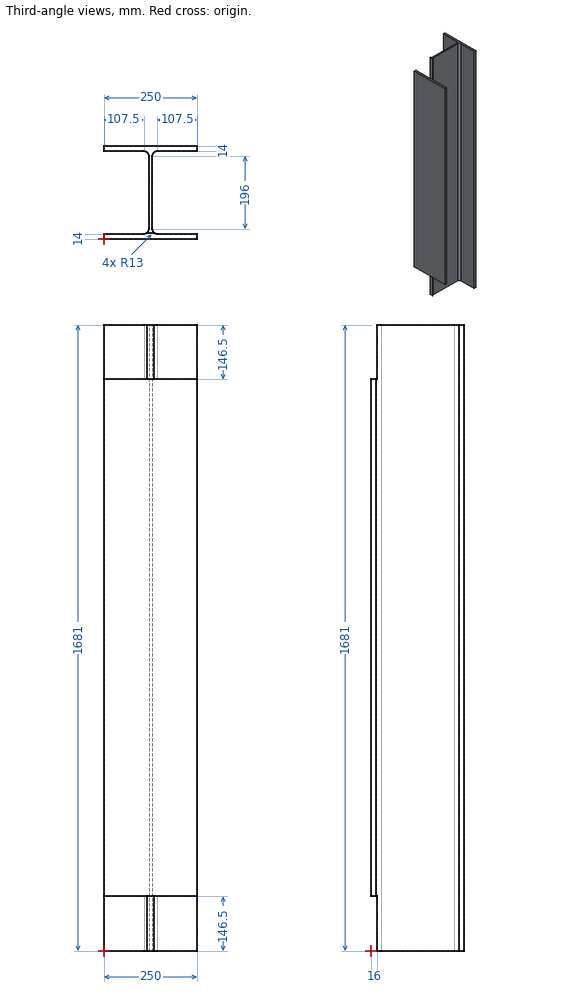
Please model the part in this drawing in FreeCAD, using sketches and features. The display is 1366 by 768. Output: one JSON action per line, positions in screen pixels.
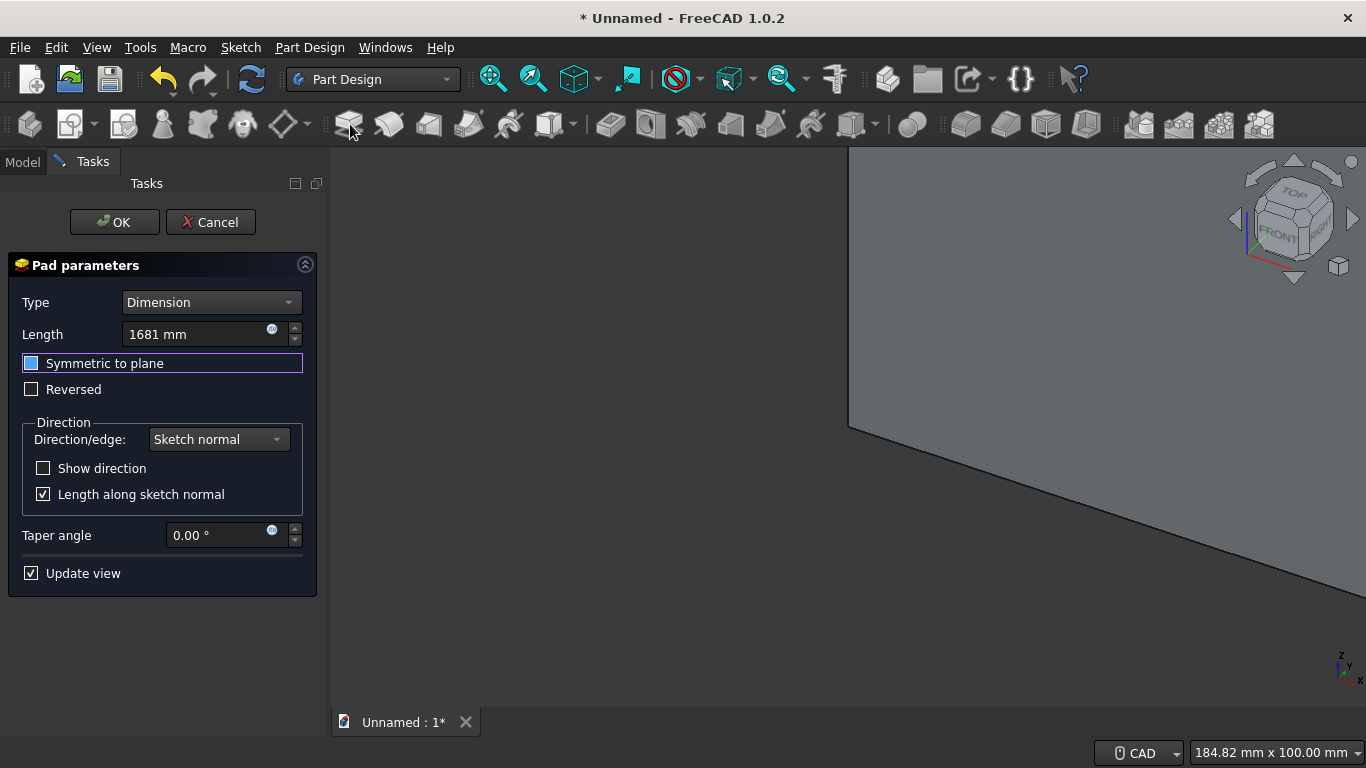
{"action": "left_click", "coordinate": [115, 222]}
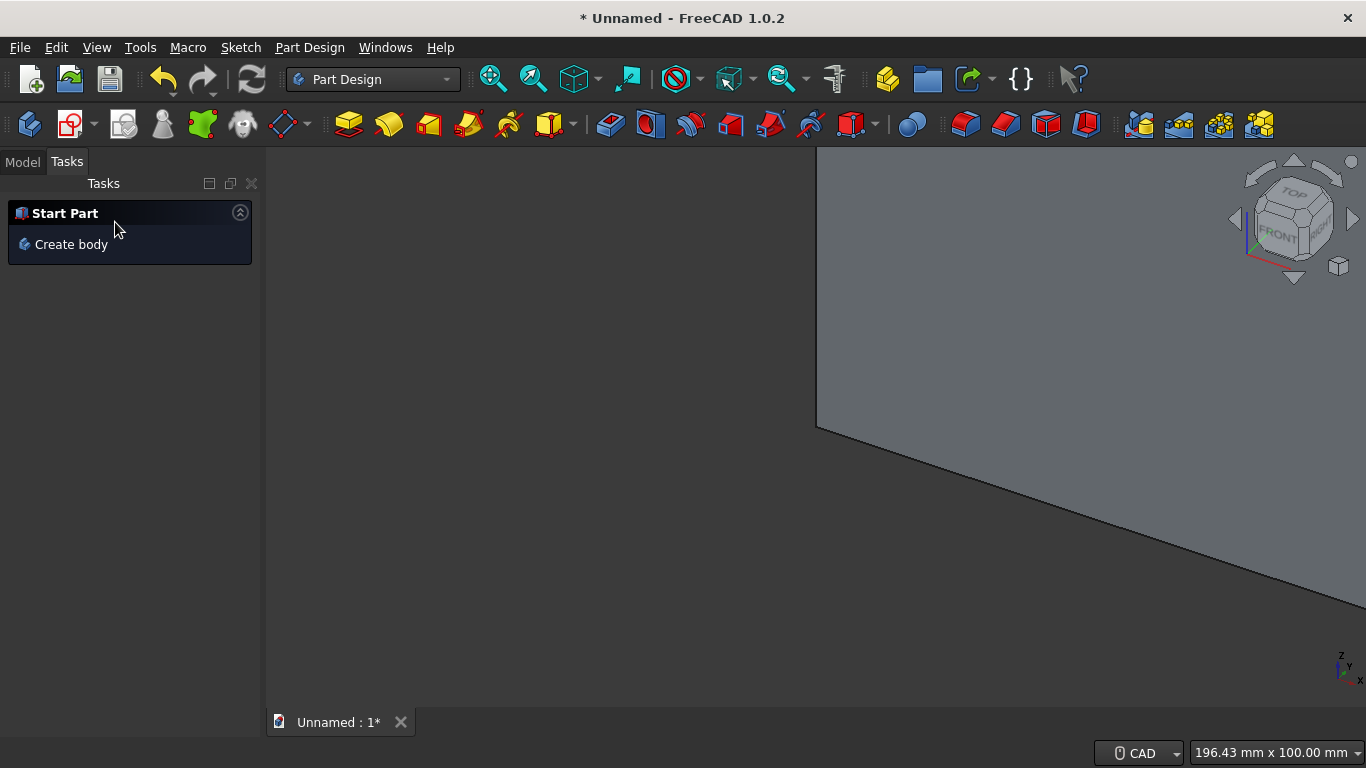
{"action": "left_click", "coordinate": [494, 80]}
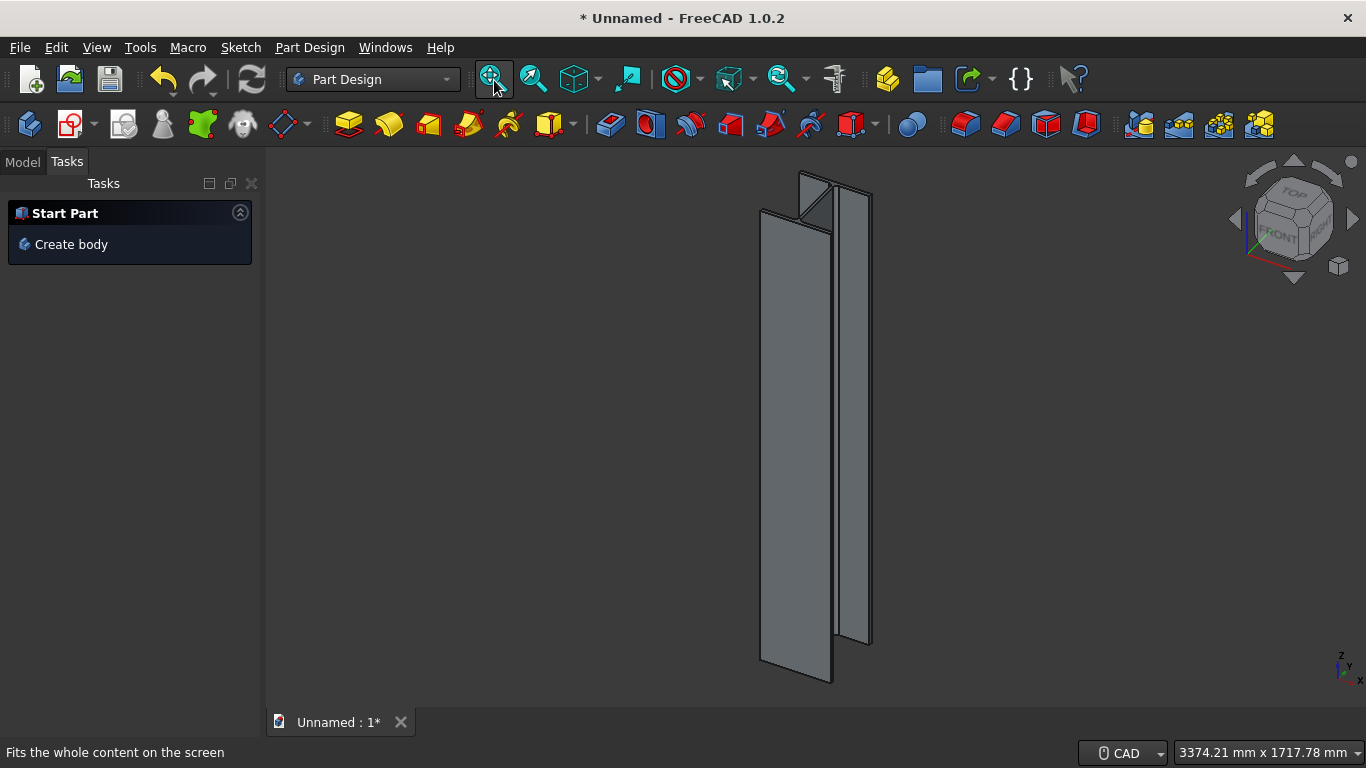
{"action": "left_click", "coordinate": [796, 318]}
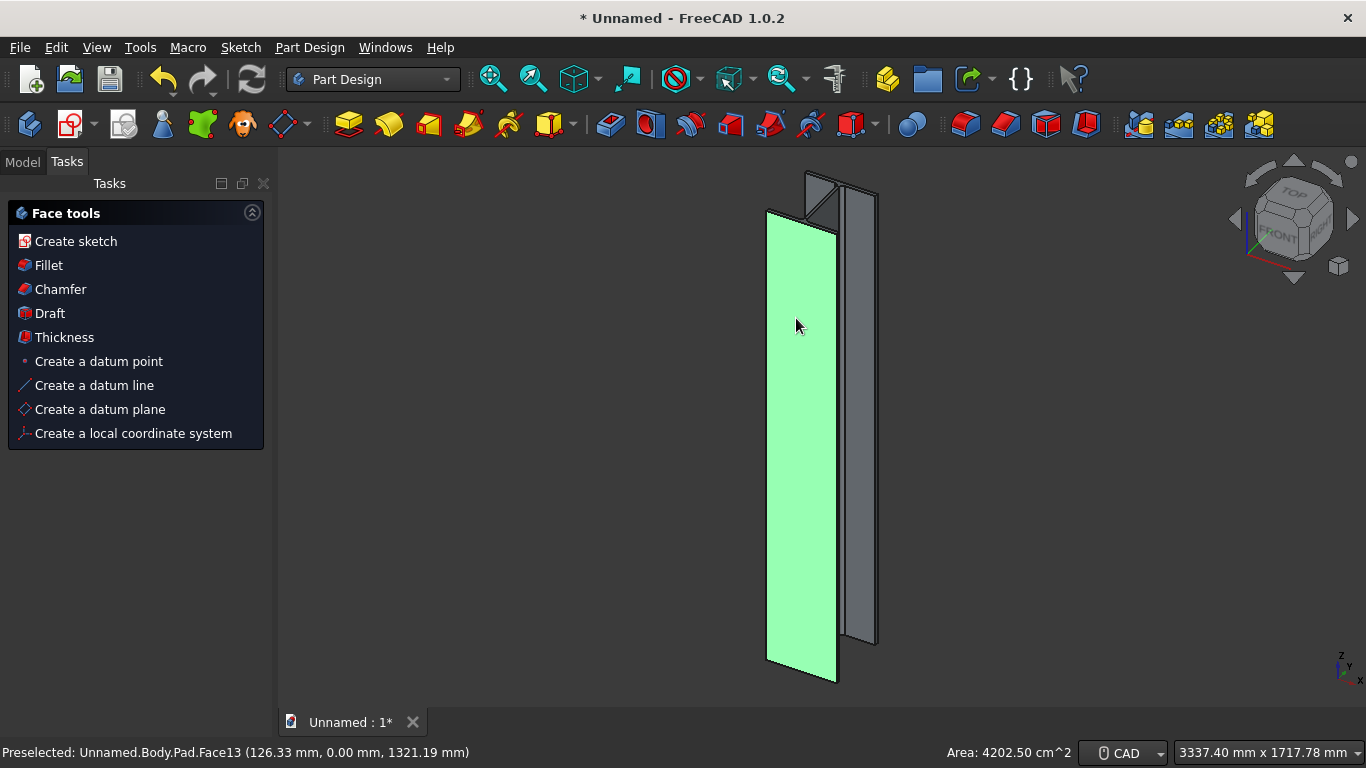
{"action": "left_click", "coordinate": [70, 124]}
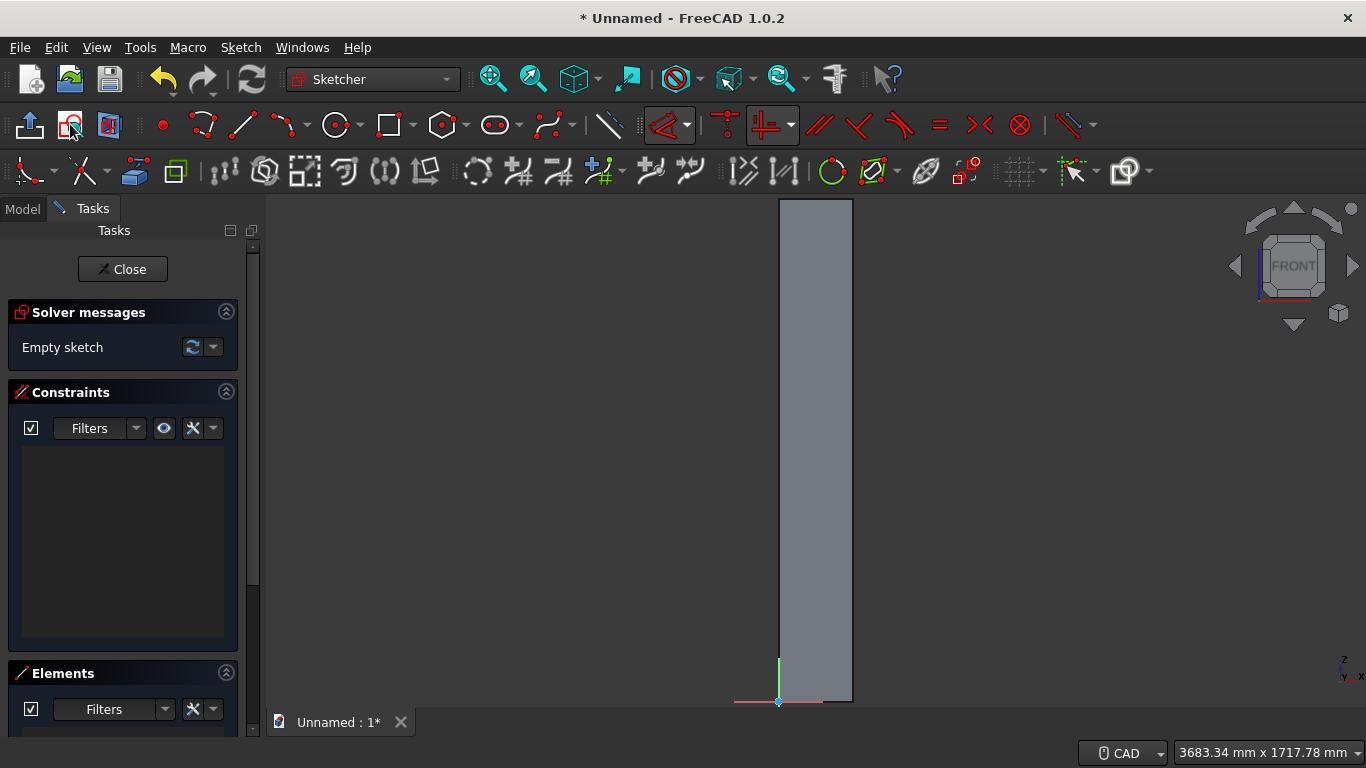
{"action": "scroll", "coordinate": [608, 451], "scroll_direction": "down", "scroll_amount": 2}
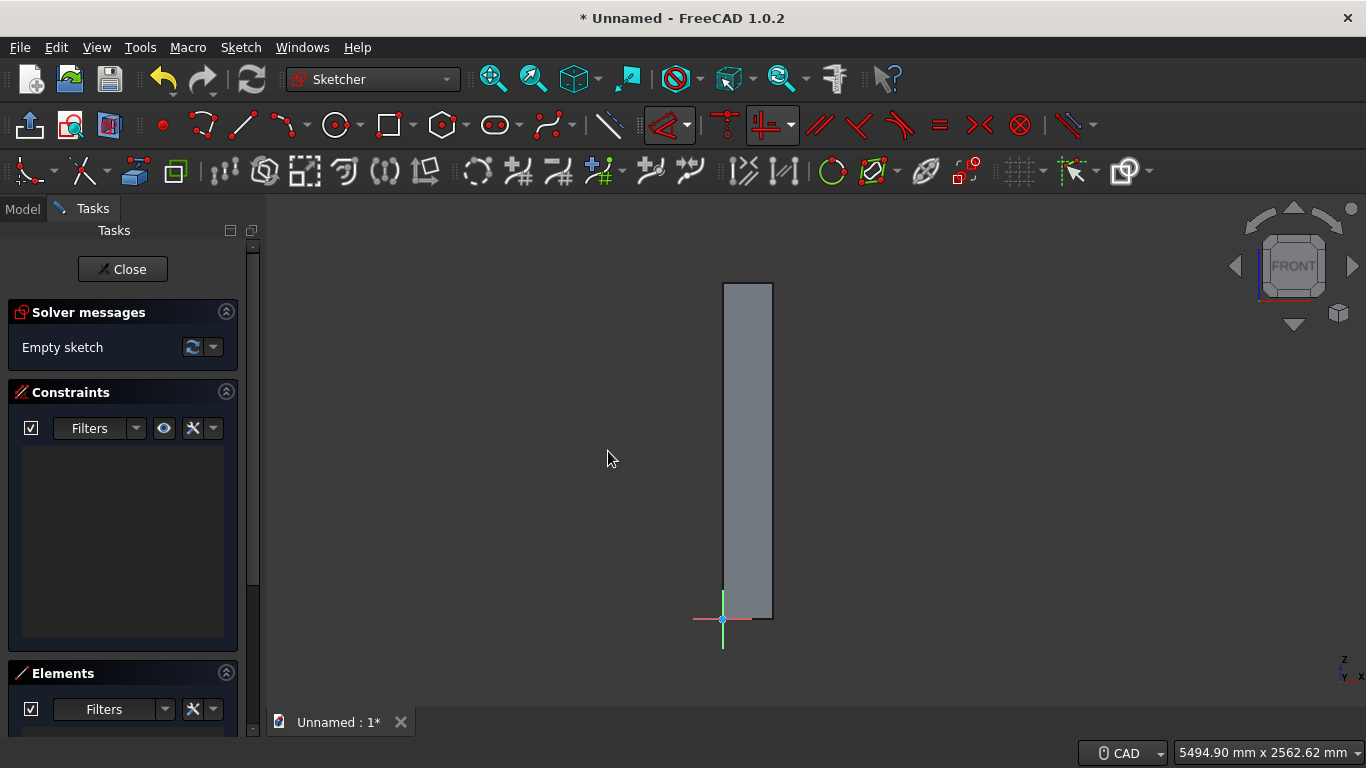
{"action": "left_click", "coordinate": [390, 126]}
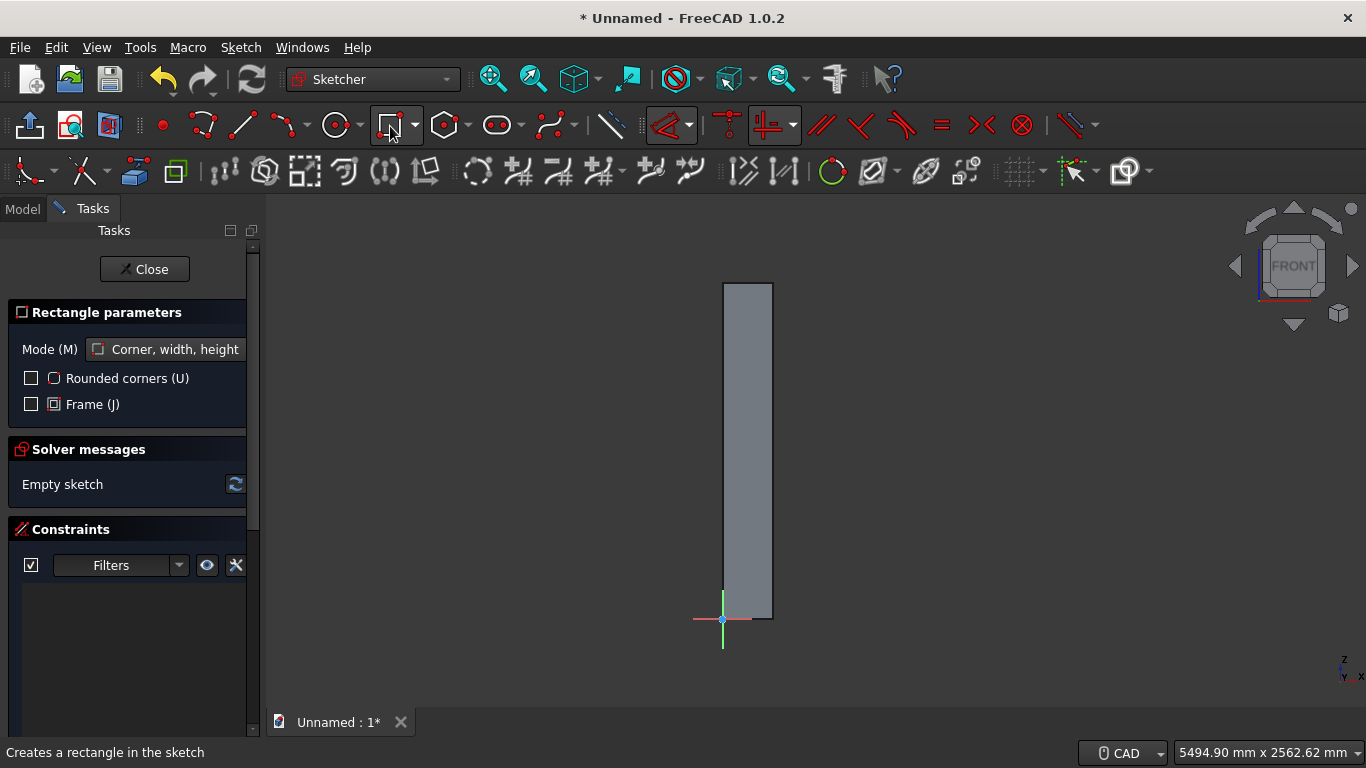
{"action": "left_click", "coordinate": [723, 619]}
{"action": "mouse_move", "coordinate": [773, 590]}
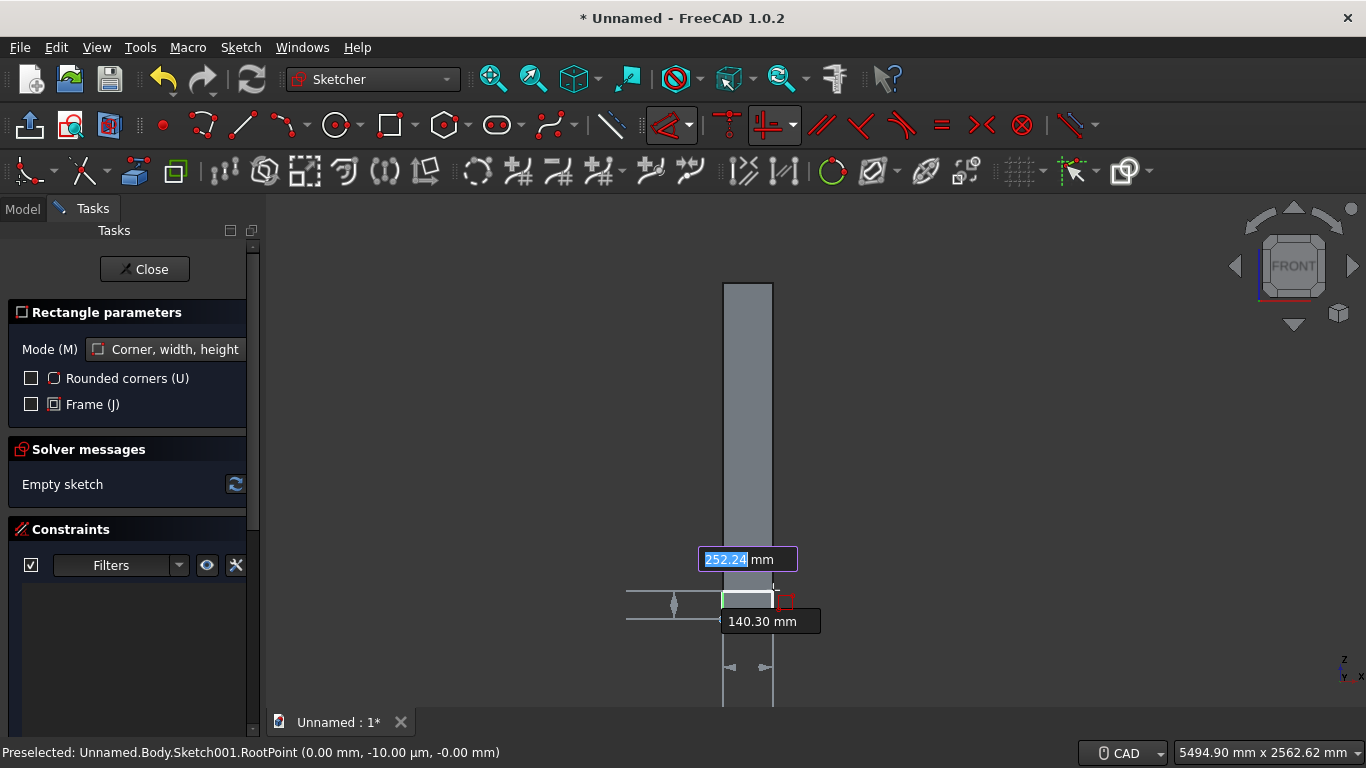
{"action": "type", "text": "250"}
{"action": "key", "text": "Tab"}
{"action": "type", "text": "146.5"}
{"action": "key", "text": "Return"}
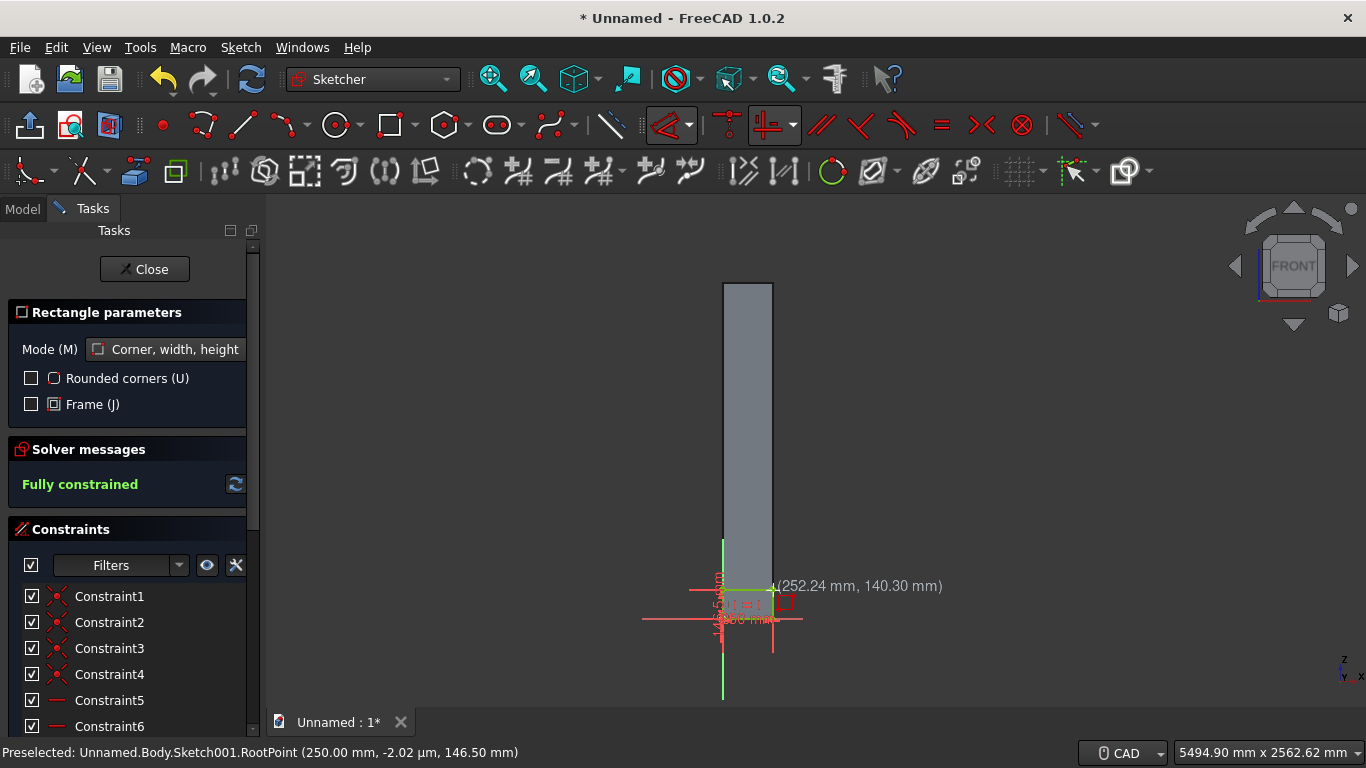
{"action": "left_click", "coordinate": [723, 283]}
{"action": "mouse_move", "coordinate": [773, 312]}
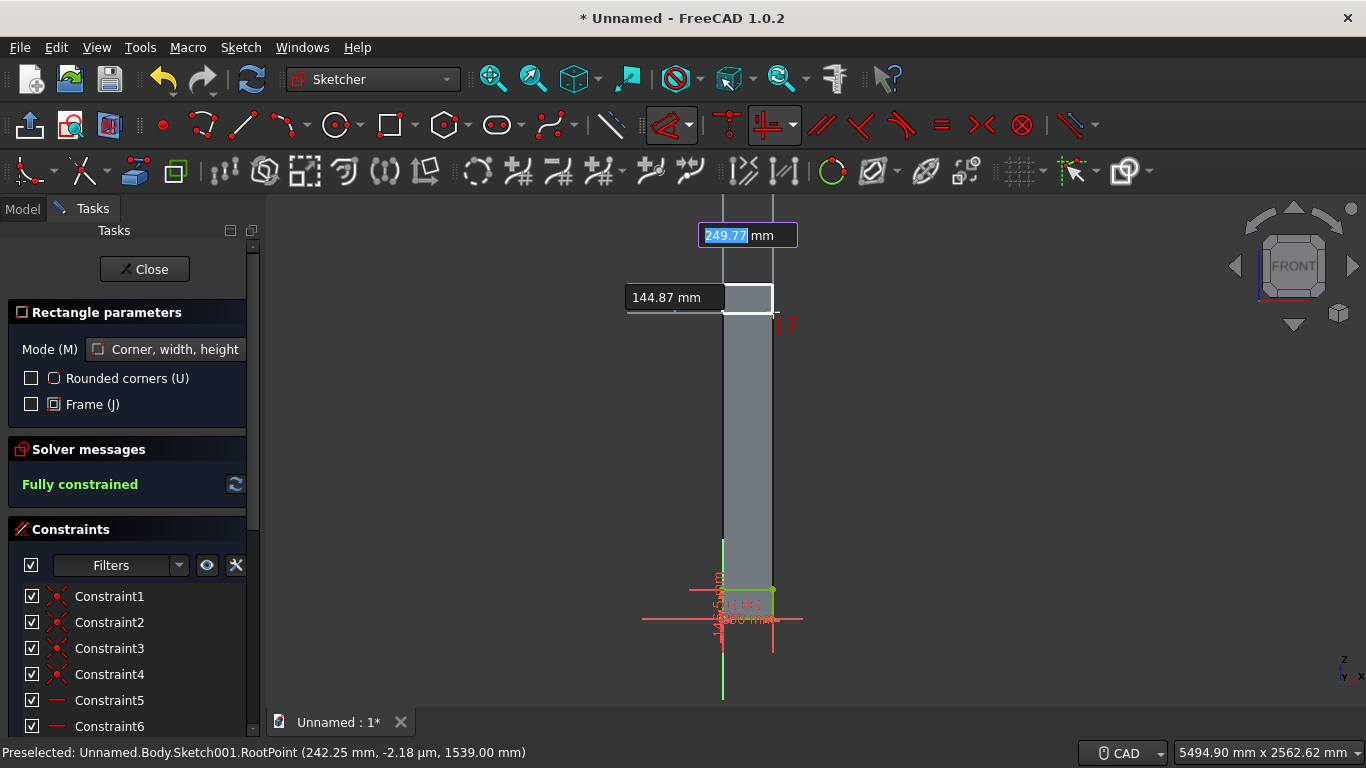
{"action": "type", "text": "250"}
{"action": "key", "text": "Tab"}
{"action": "type", "text": "146.5"}
{"action": "key", "text": "Return"}
{"action": "key", "text": "Escape"}